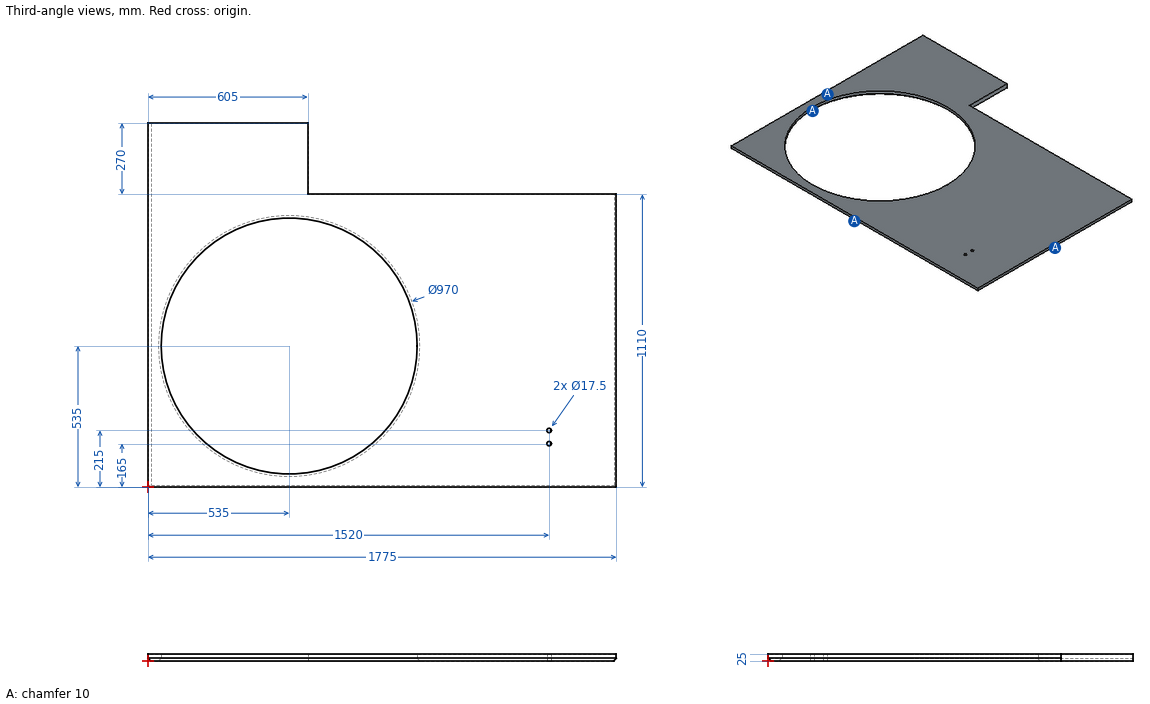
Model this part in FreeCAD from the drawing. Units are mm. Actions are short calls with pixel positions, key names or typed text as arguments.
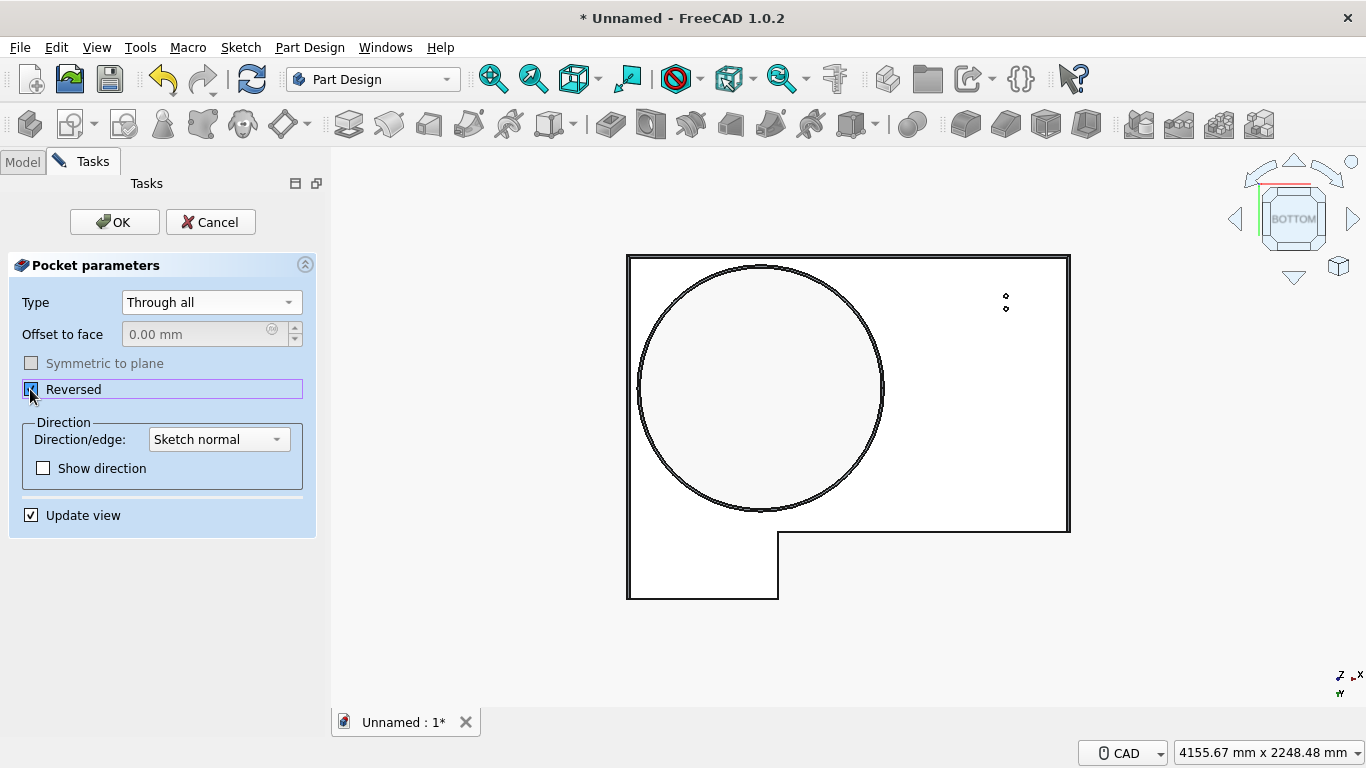
click(115, 222)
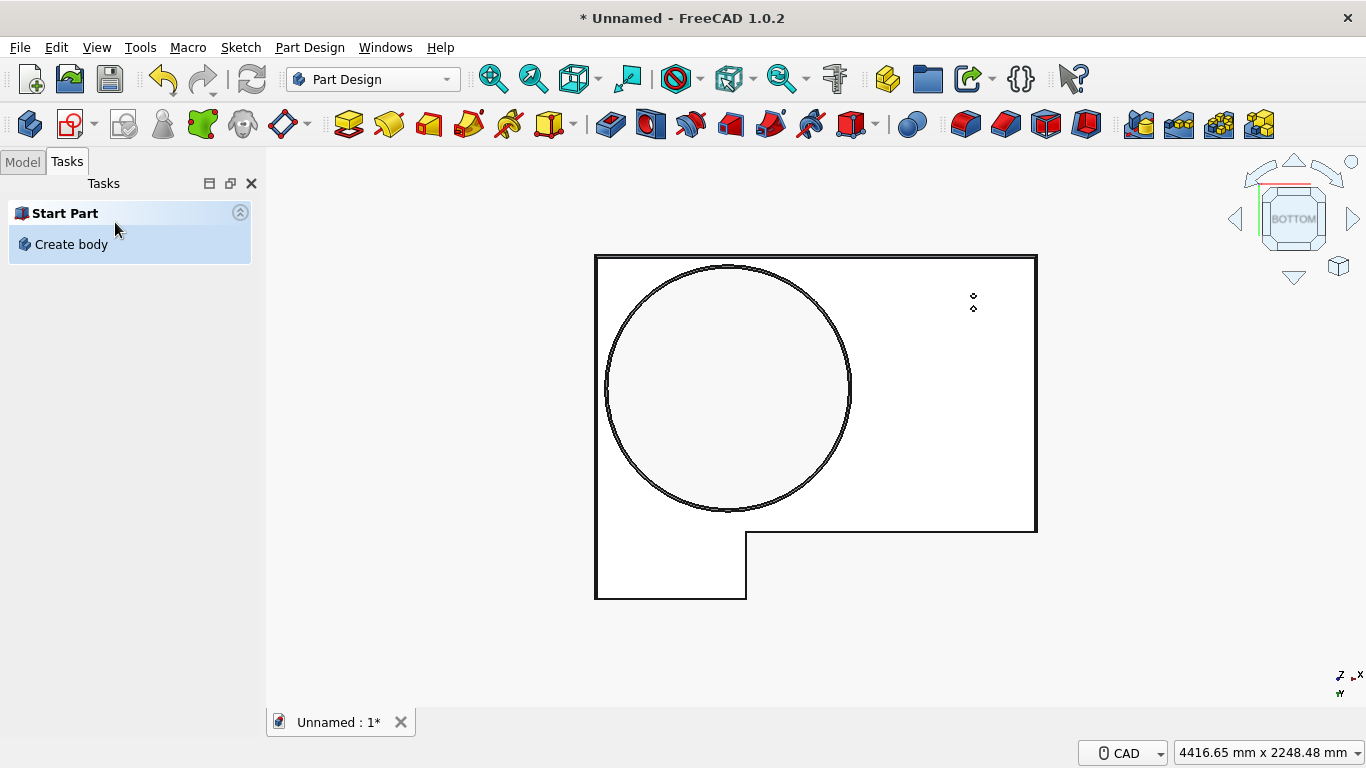
key(0)